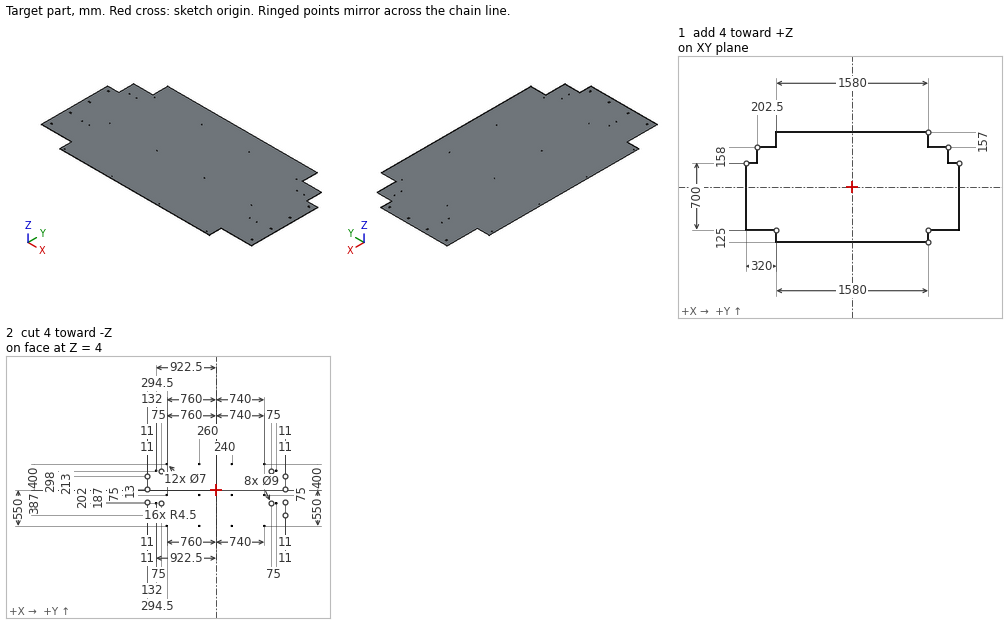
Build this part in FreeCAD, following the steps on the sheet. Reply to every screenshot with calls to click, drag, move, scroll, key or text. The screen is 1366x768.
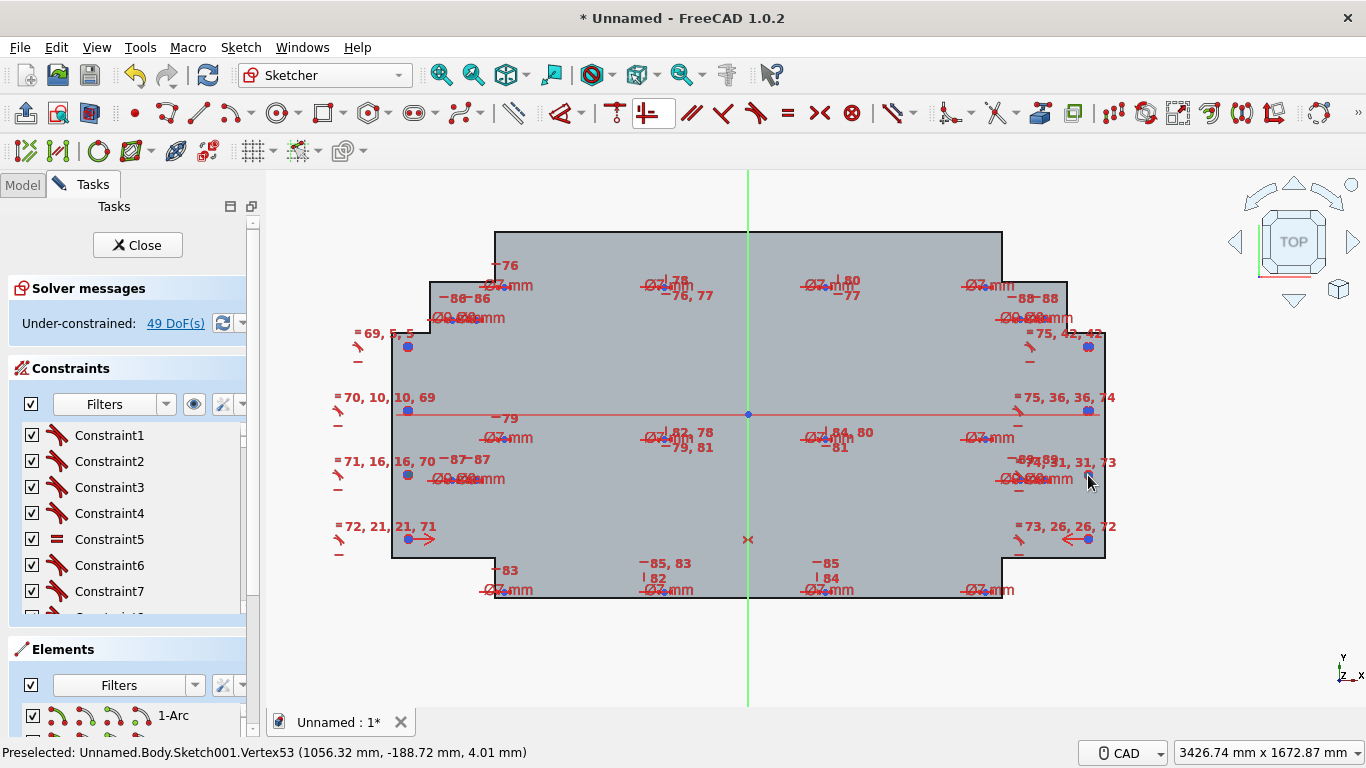
click(748, 645)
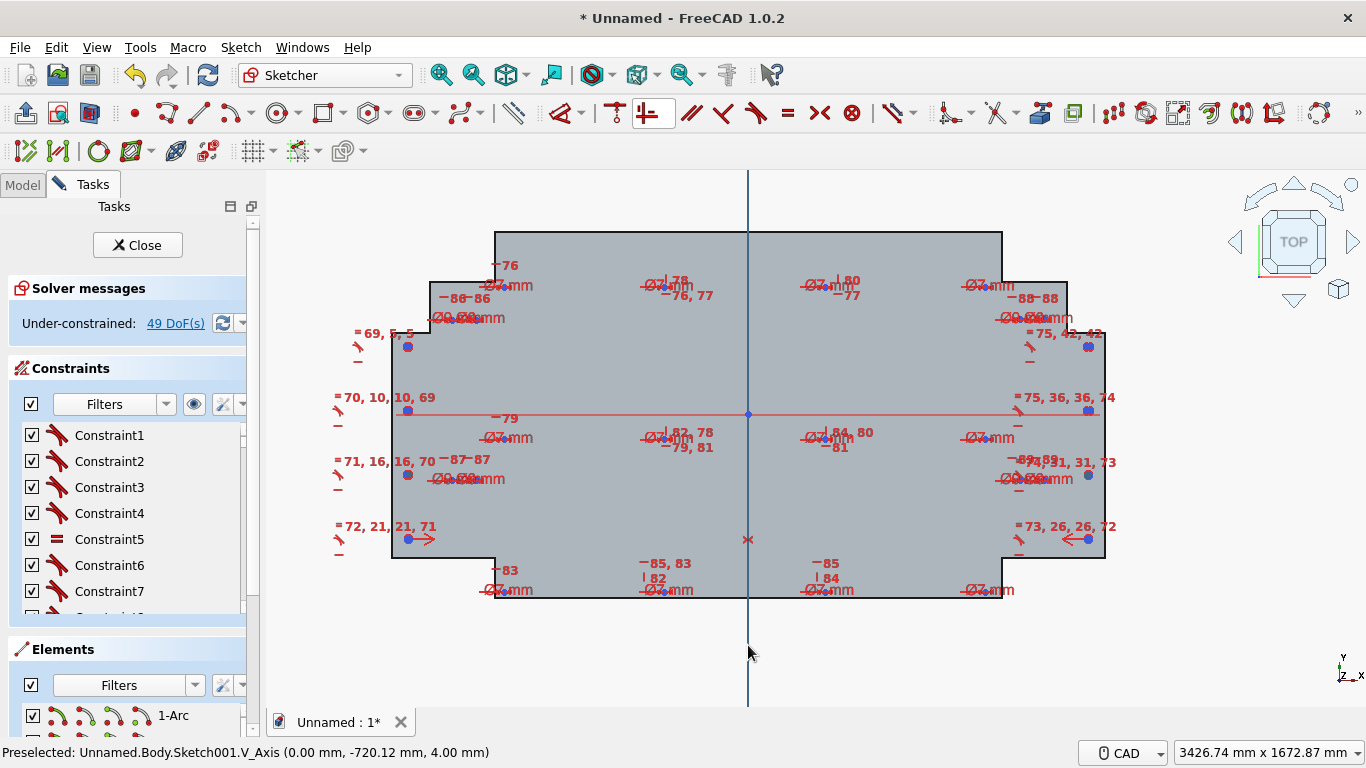
click(820, 114)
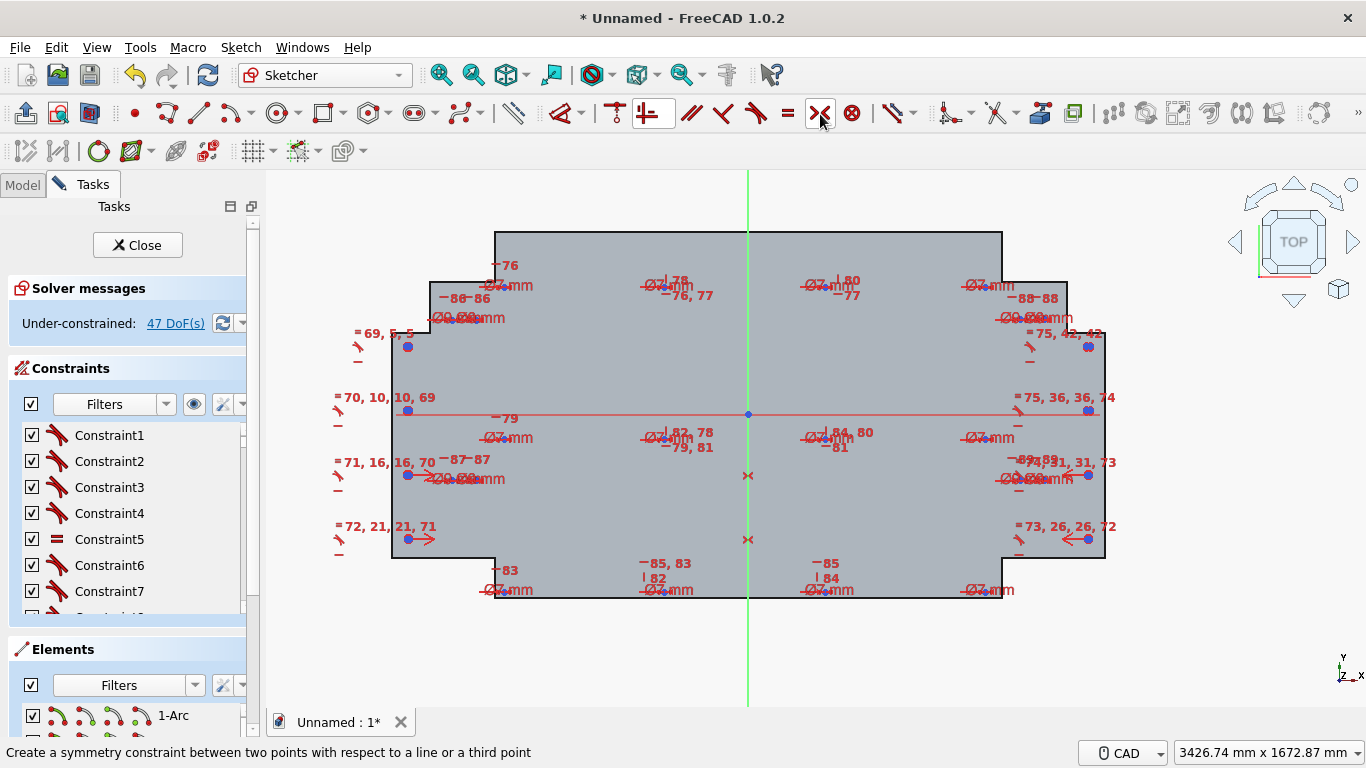
scroll(410, 411, up, 11)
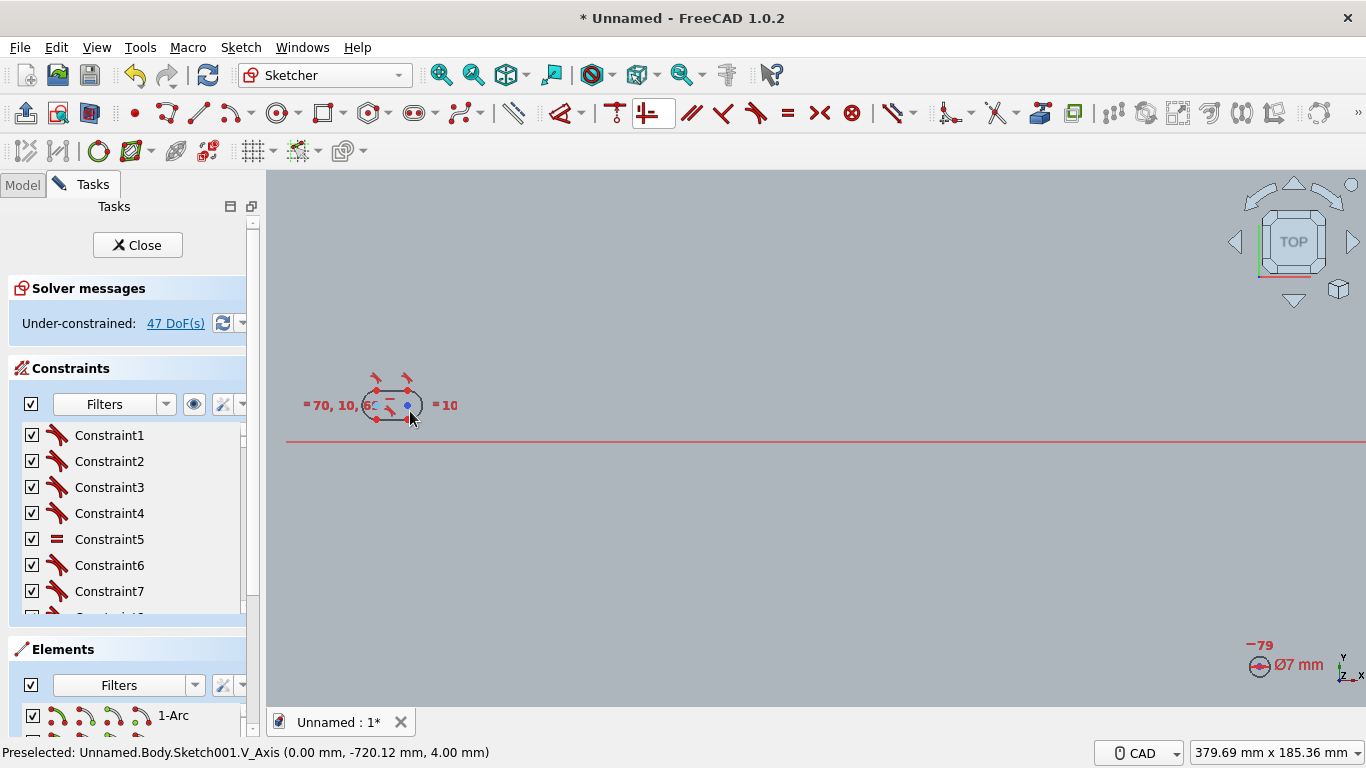
click(408, 405)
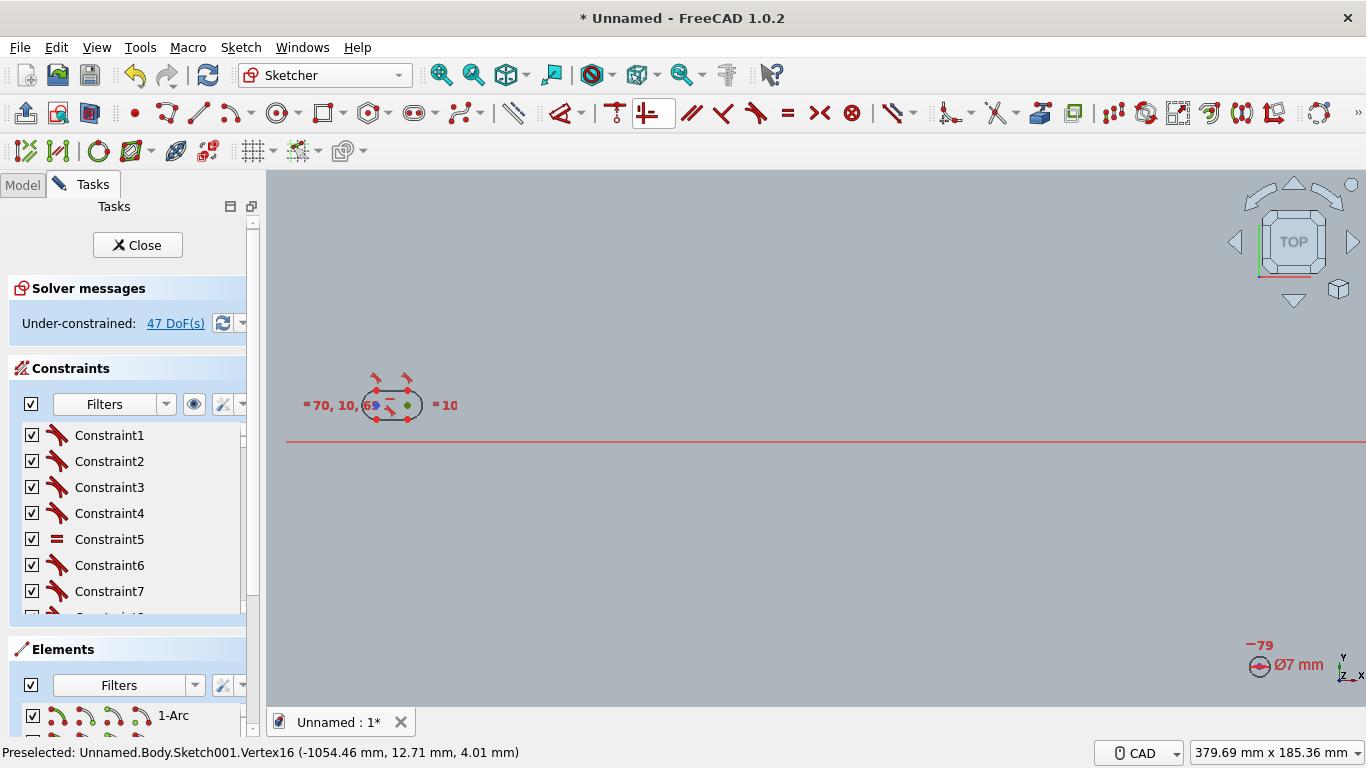
scroll(409, 411, down, 11)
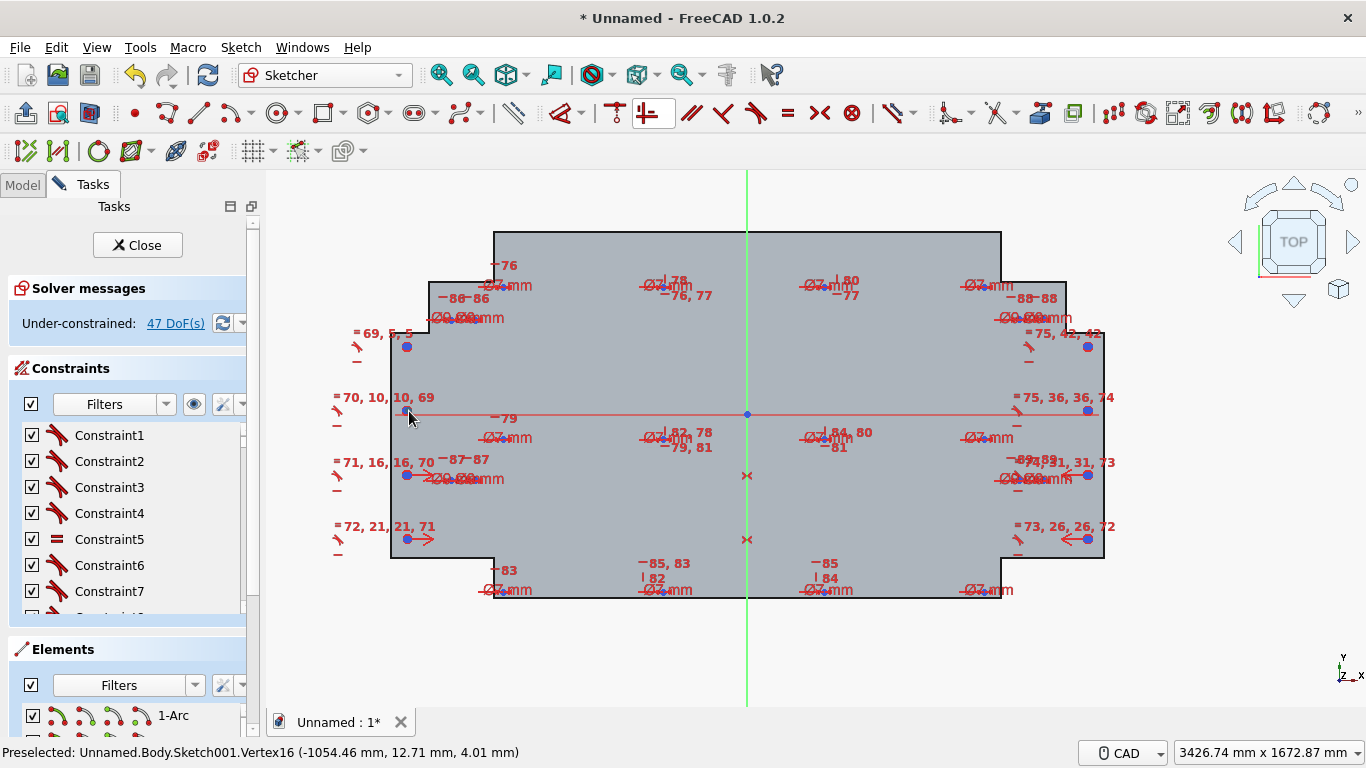
scroll(1086, 411, up, 11)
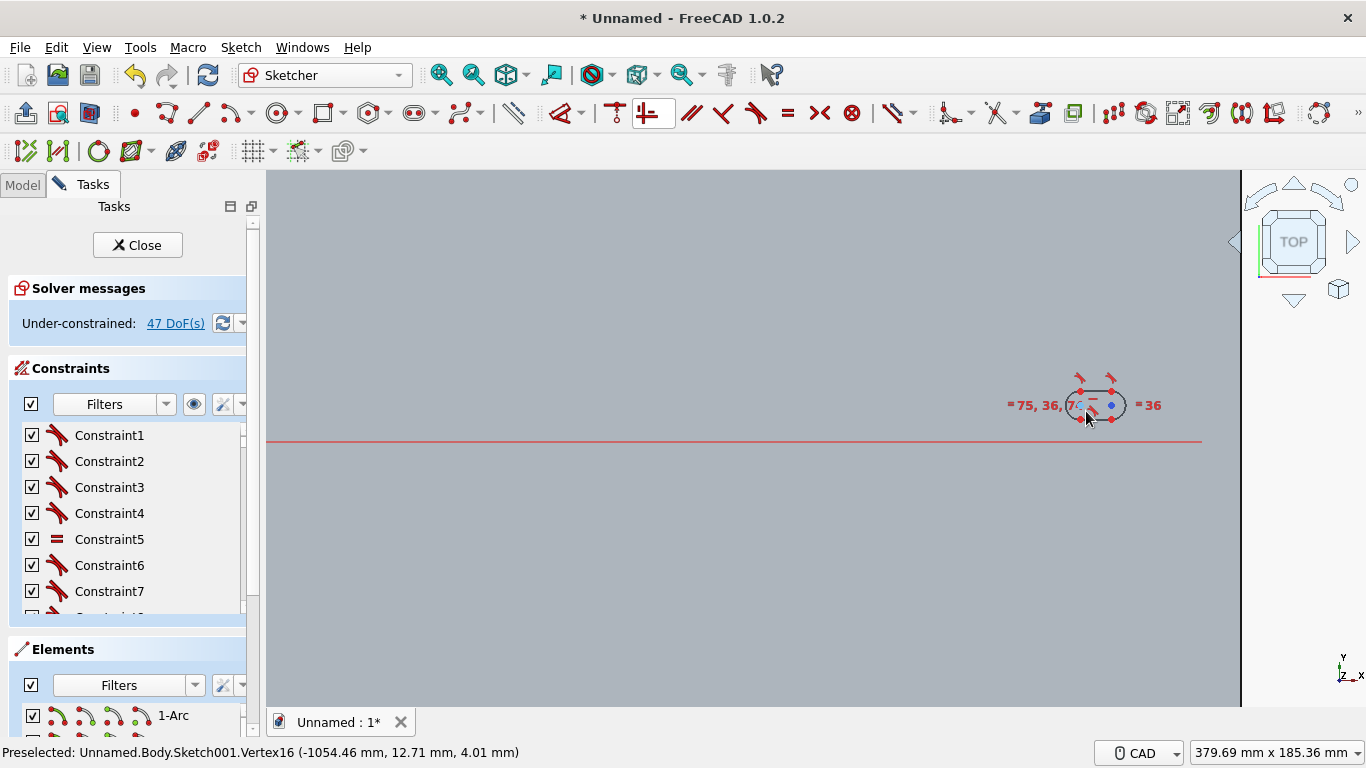
click(1080, 406)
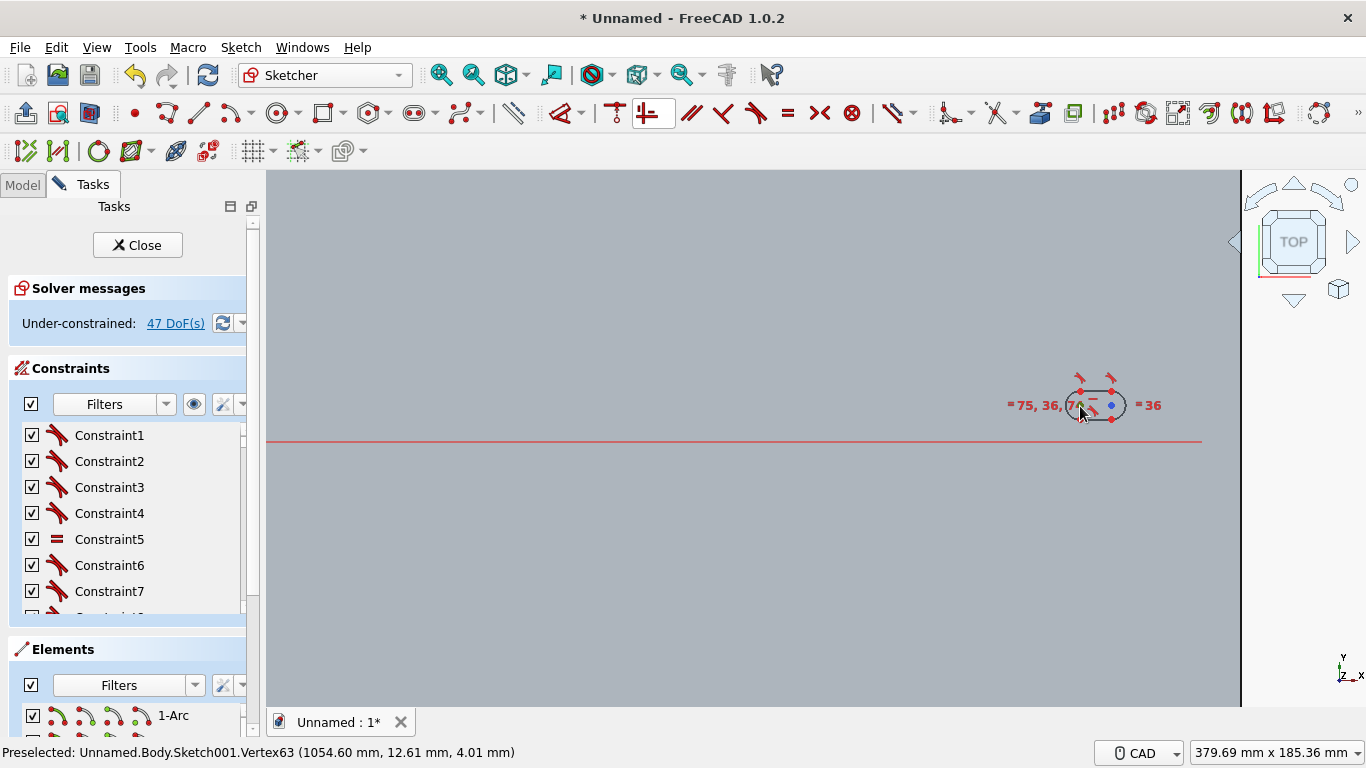
scroll(1087, 411, down, 11)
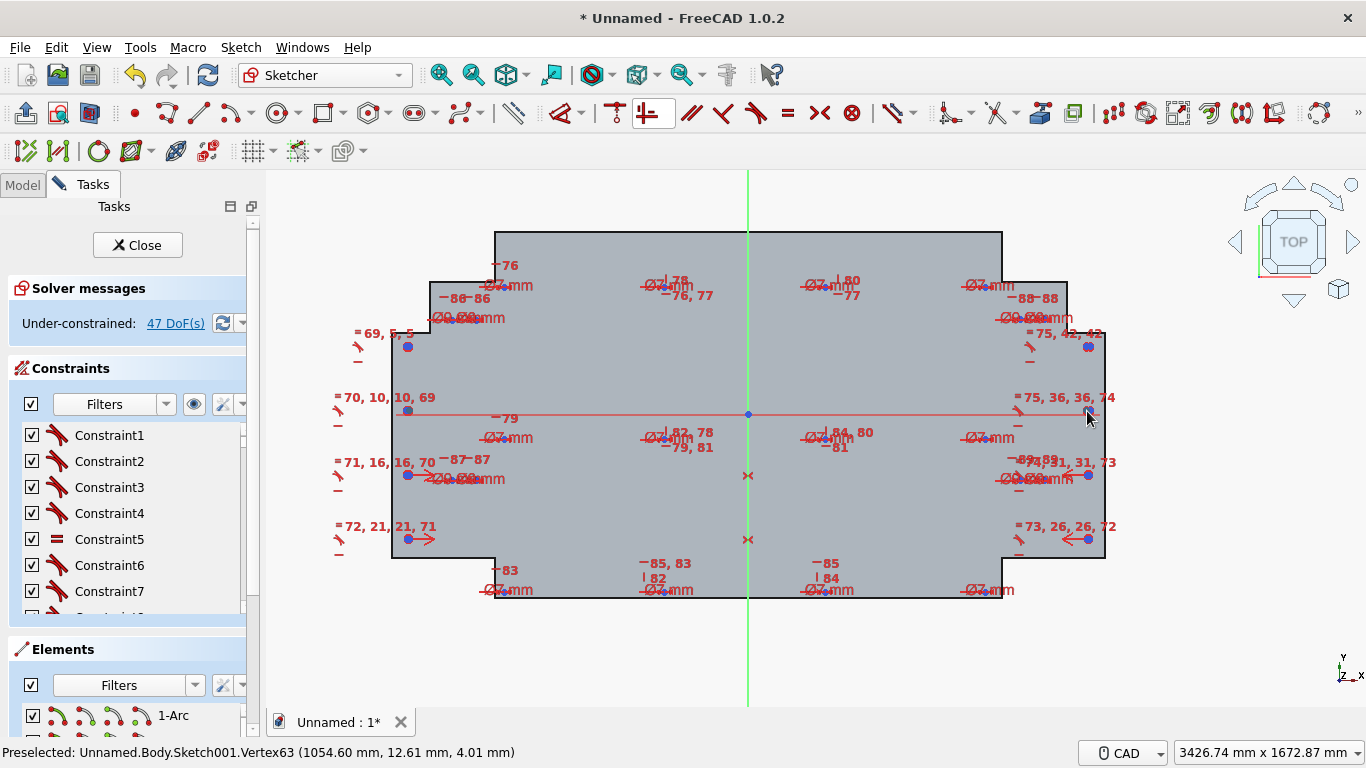
click(748, 645)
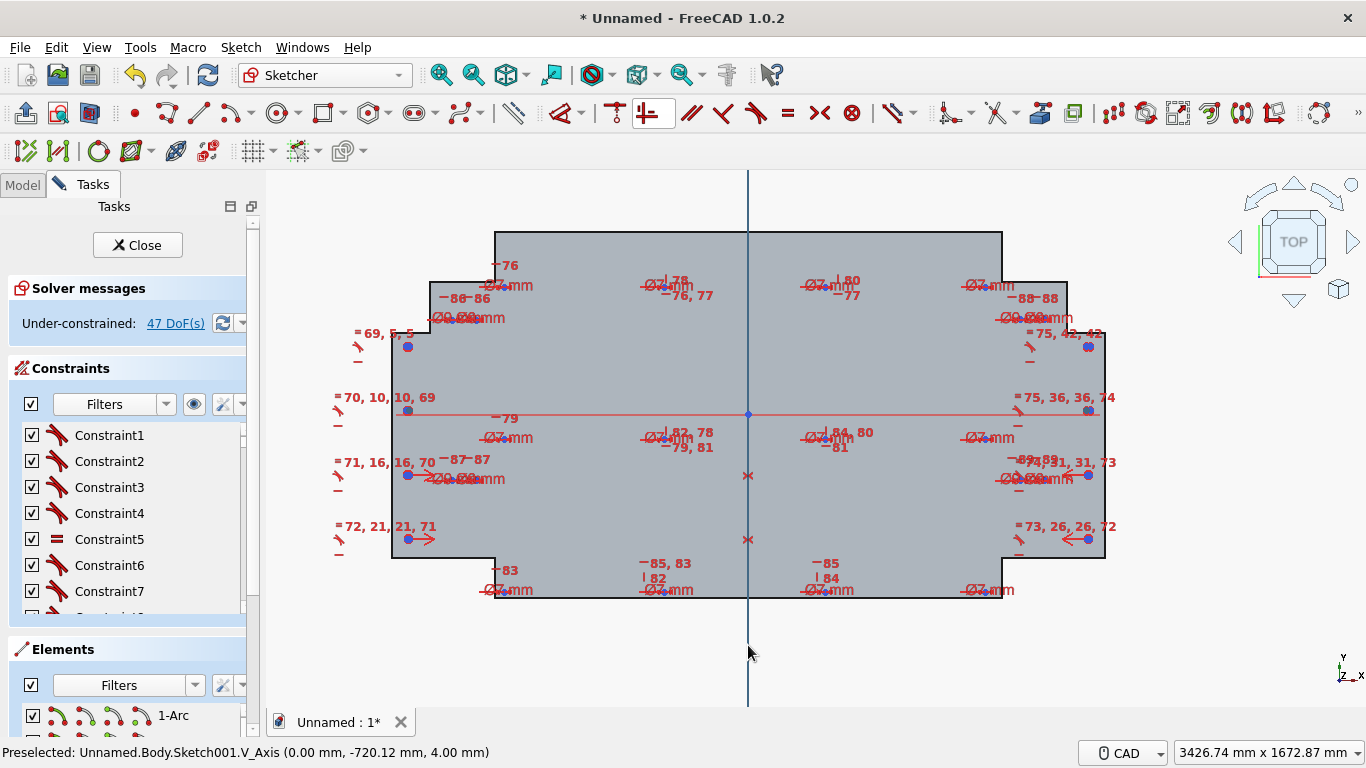
click(820, 114)